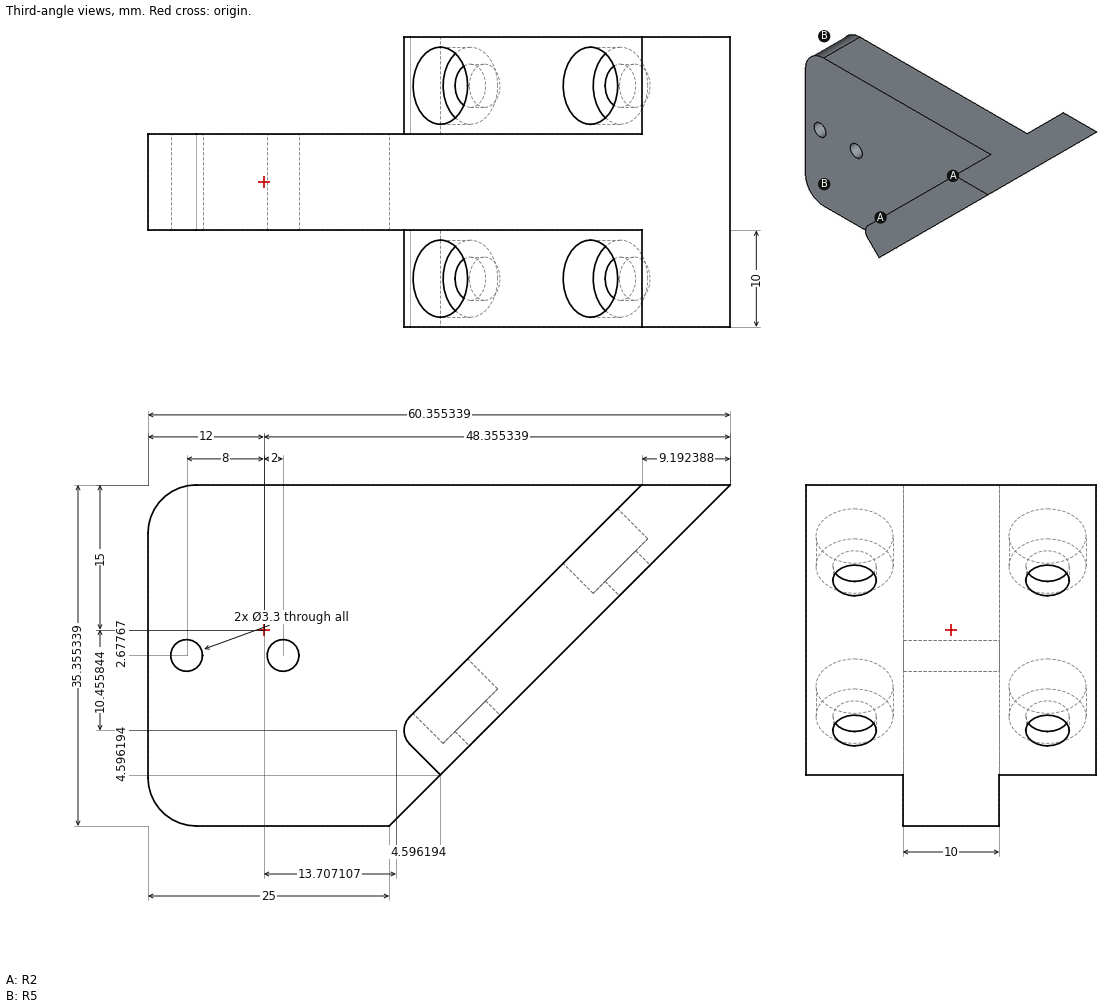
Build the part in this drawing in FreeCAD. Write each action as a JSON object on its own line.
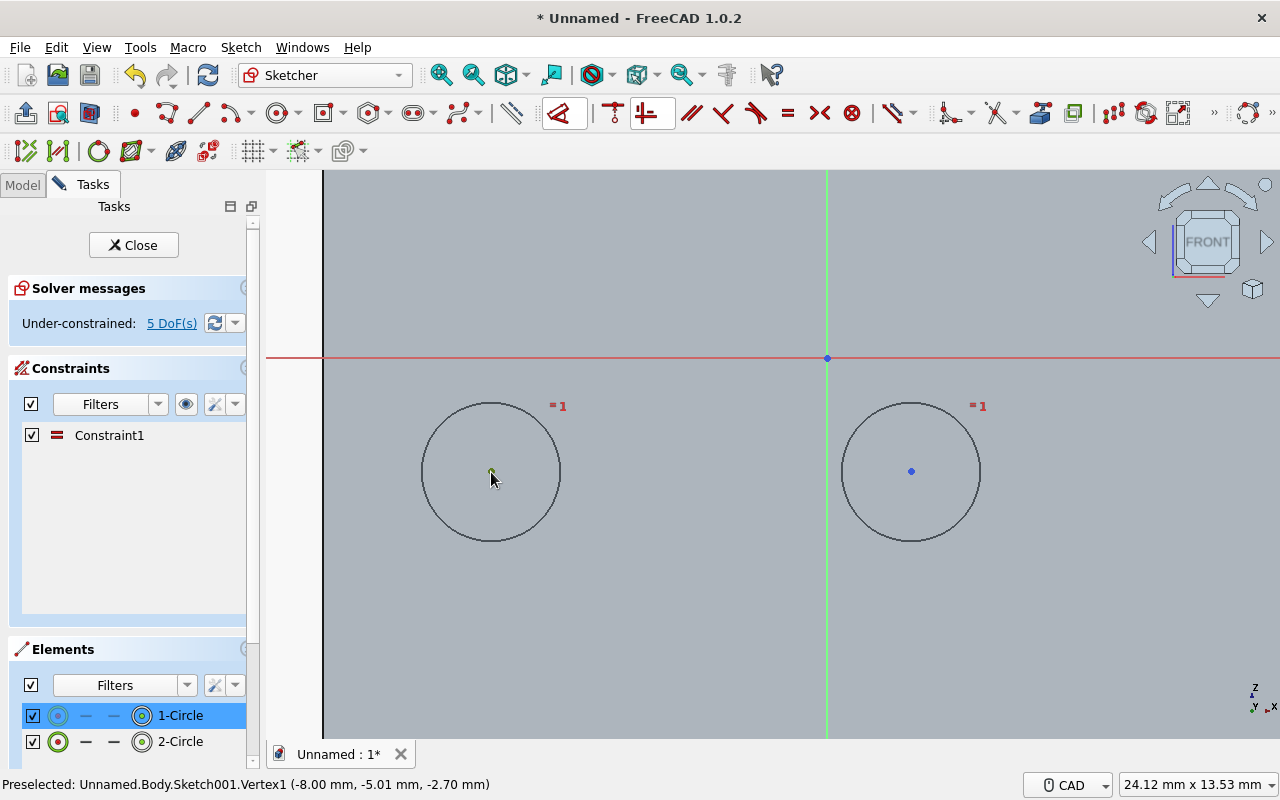
{"action": "left_click", "coordinate": [911, 472]}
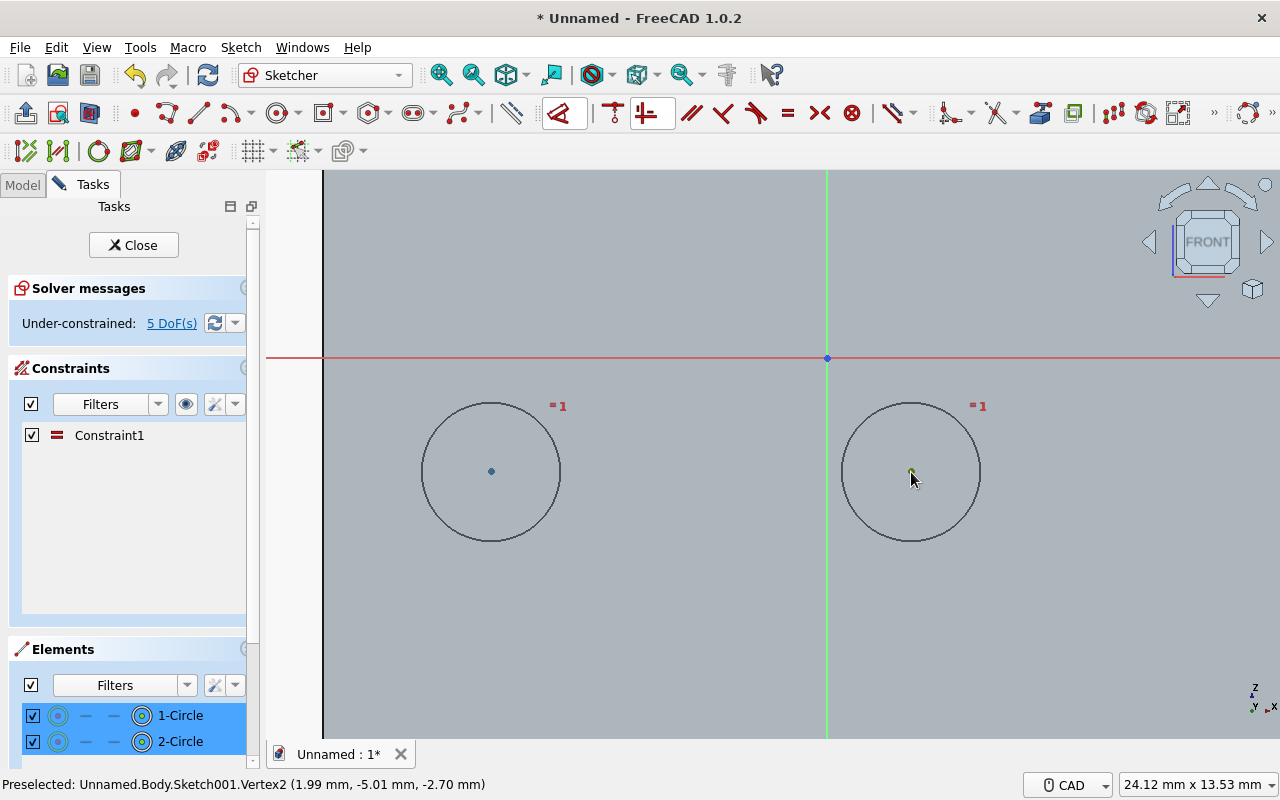
{"action": "left_click", "coordinate": [670, 114]}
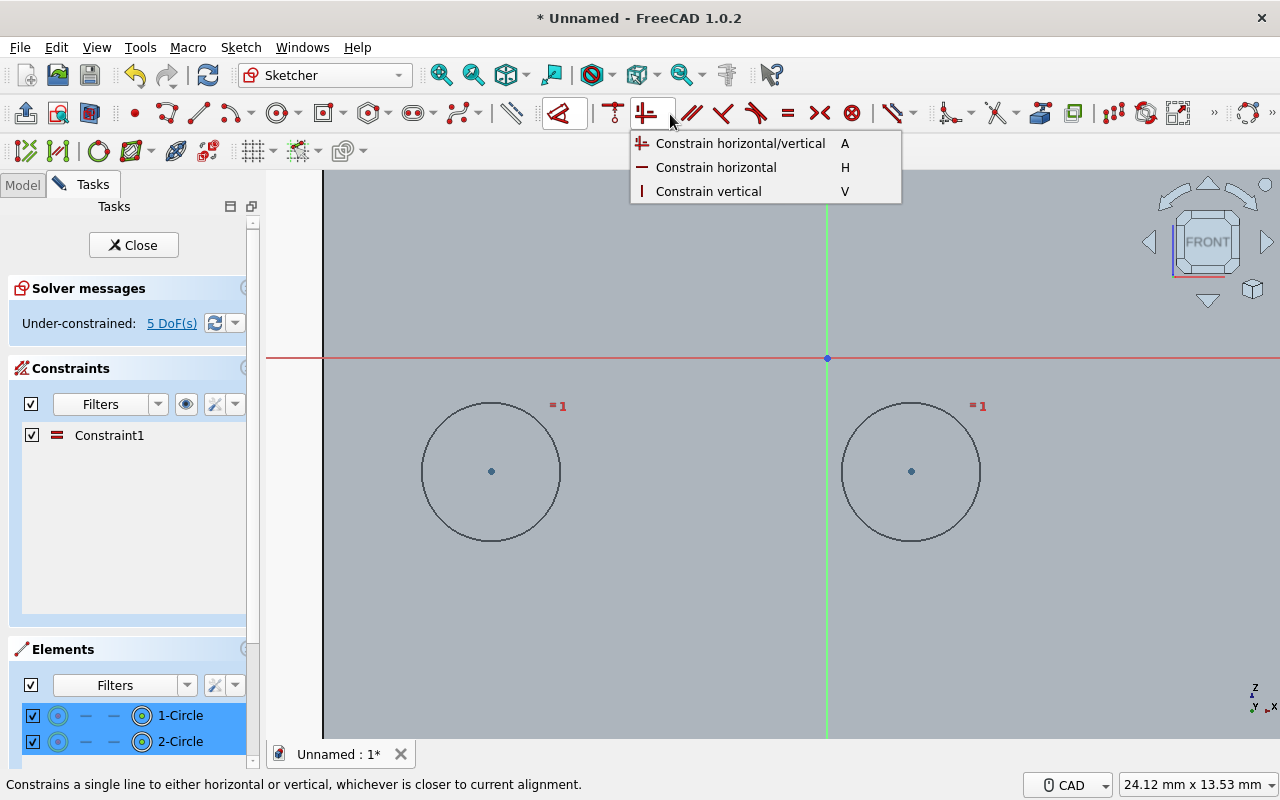
{"action": "left_click", "coordinate": [766, 167]}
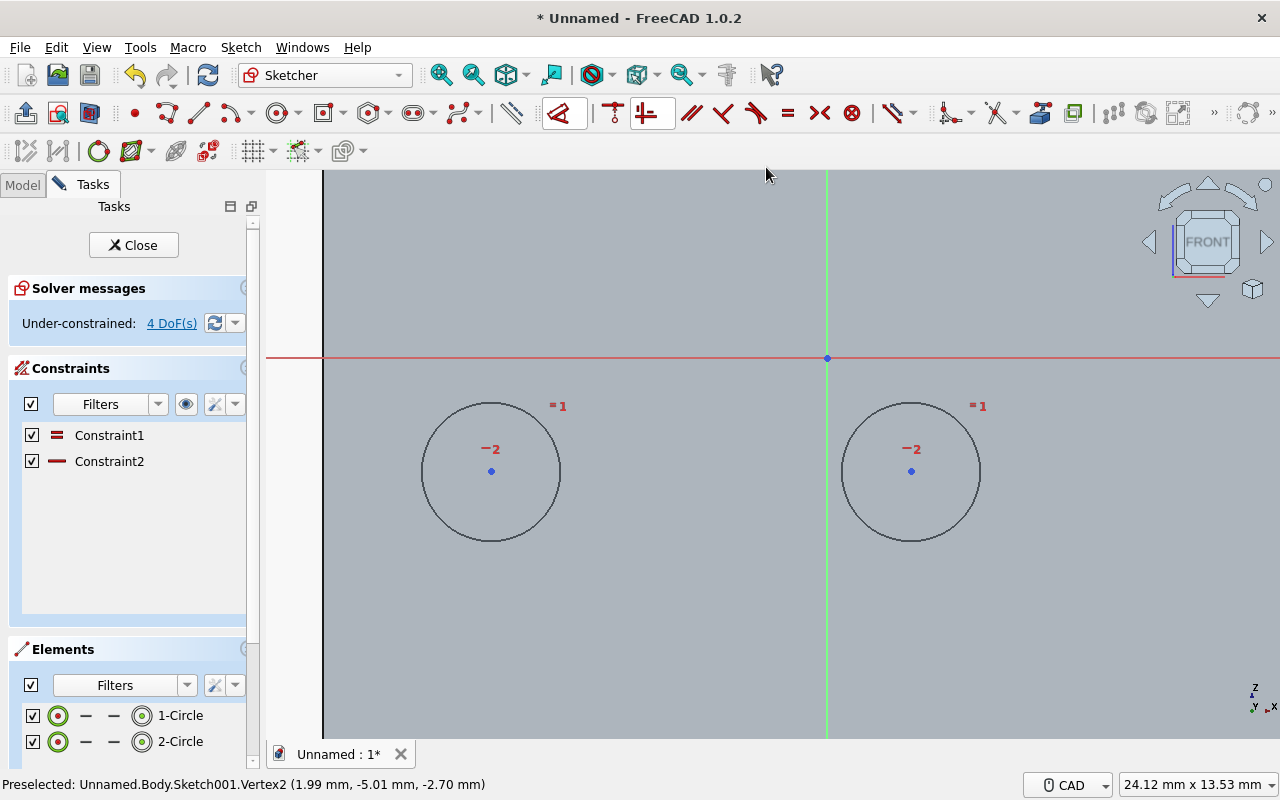
{"action": "left_click", "coordinate": [540, 423]}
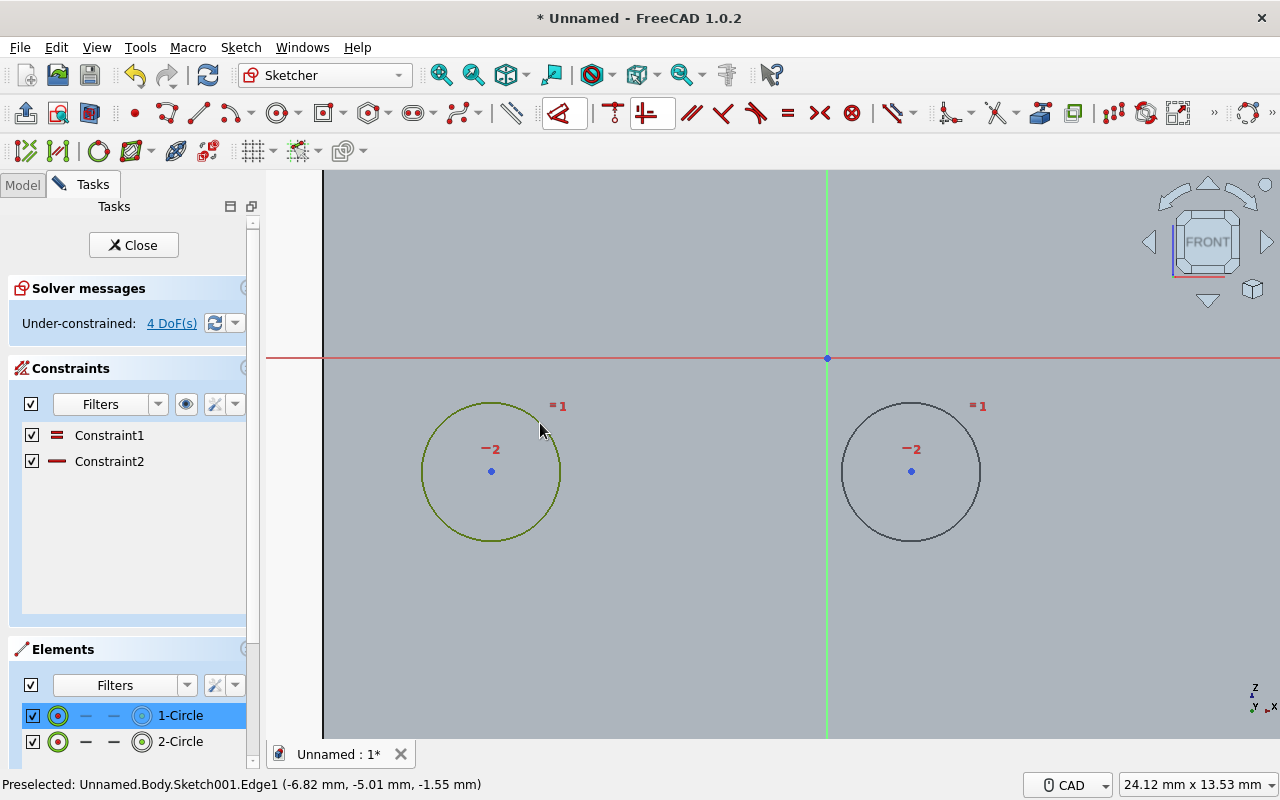
{"action": "left_click", "coordinate": [582, 114]}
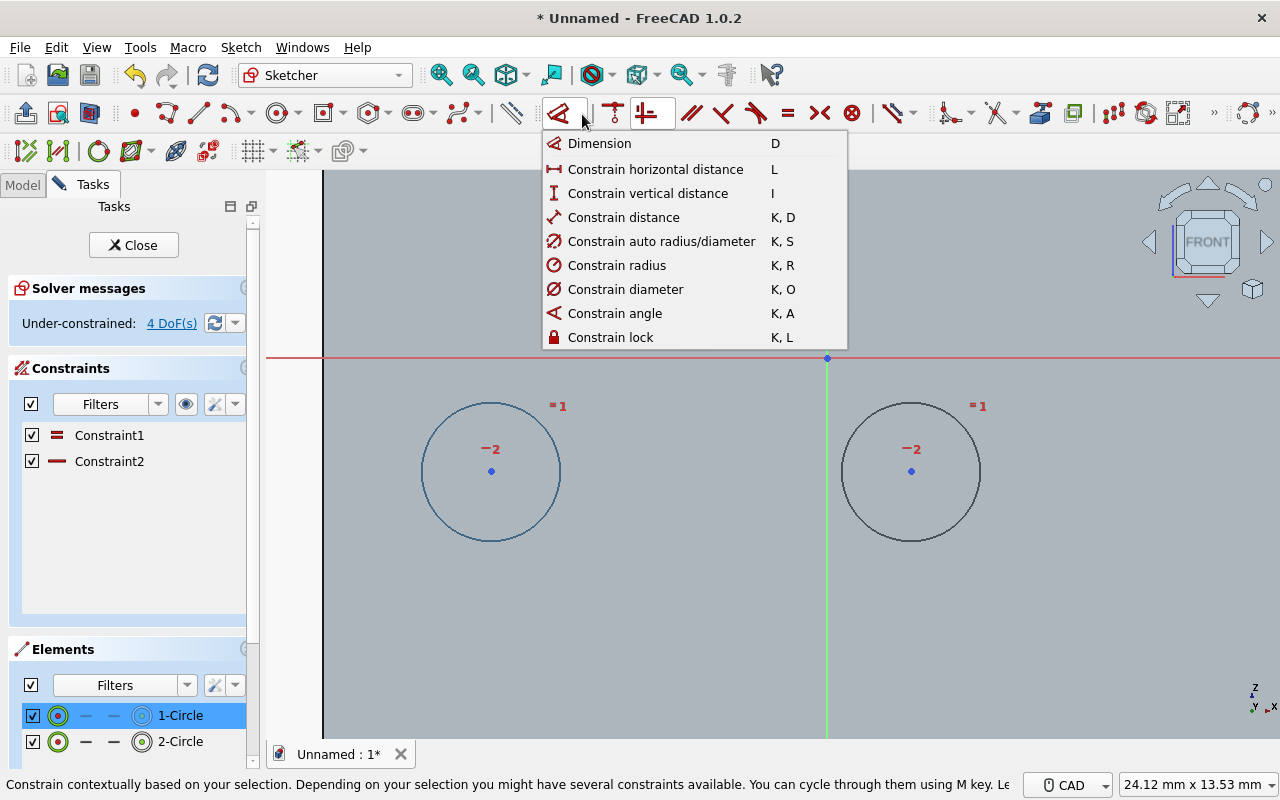
{"action": "left_click", "coordinate": [695, 289]}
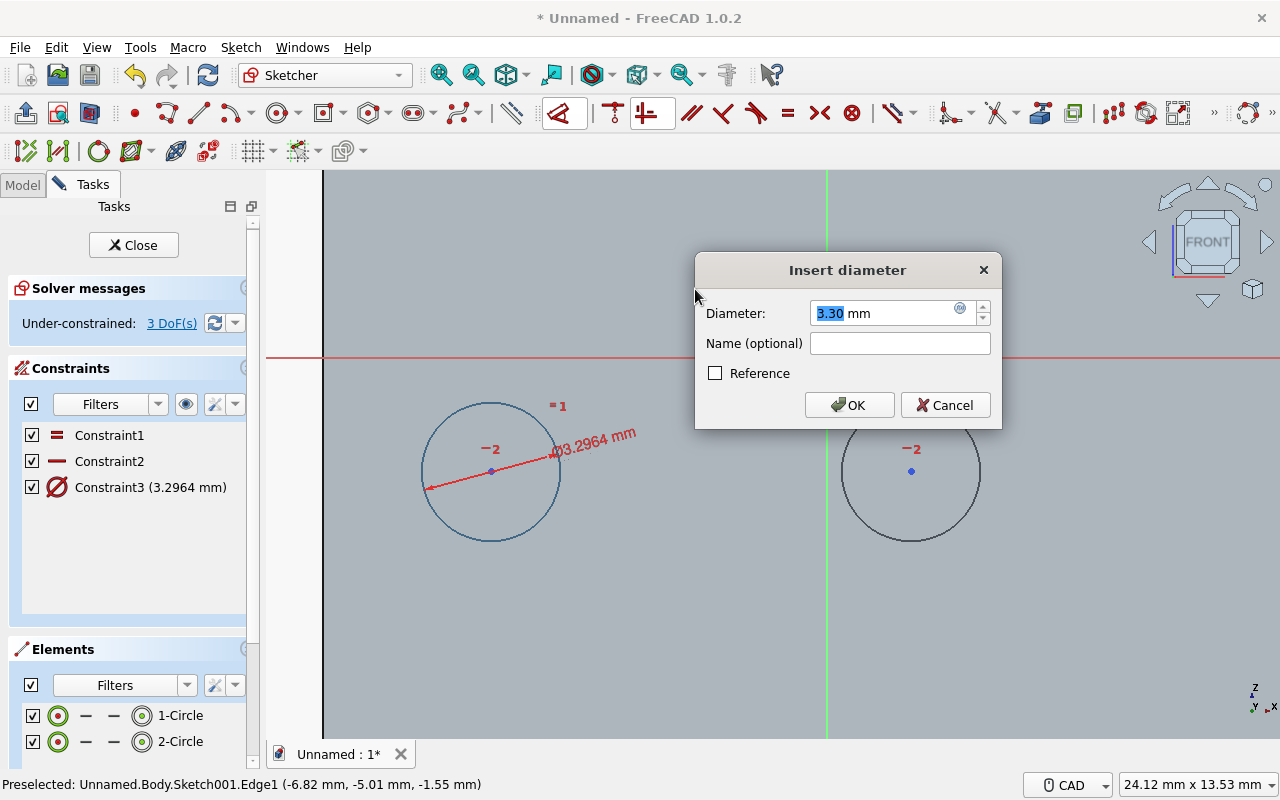
{"action": "type", "text": "3.3"}
{"action": "key", "text": "Return"}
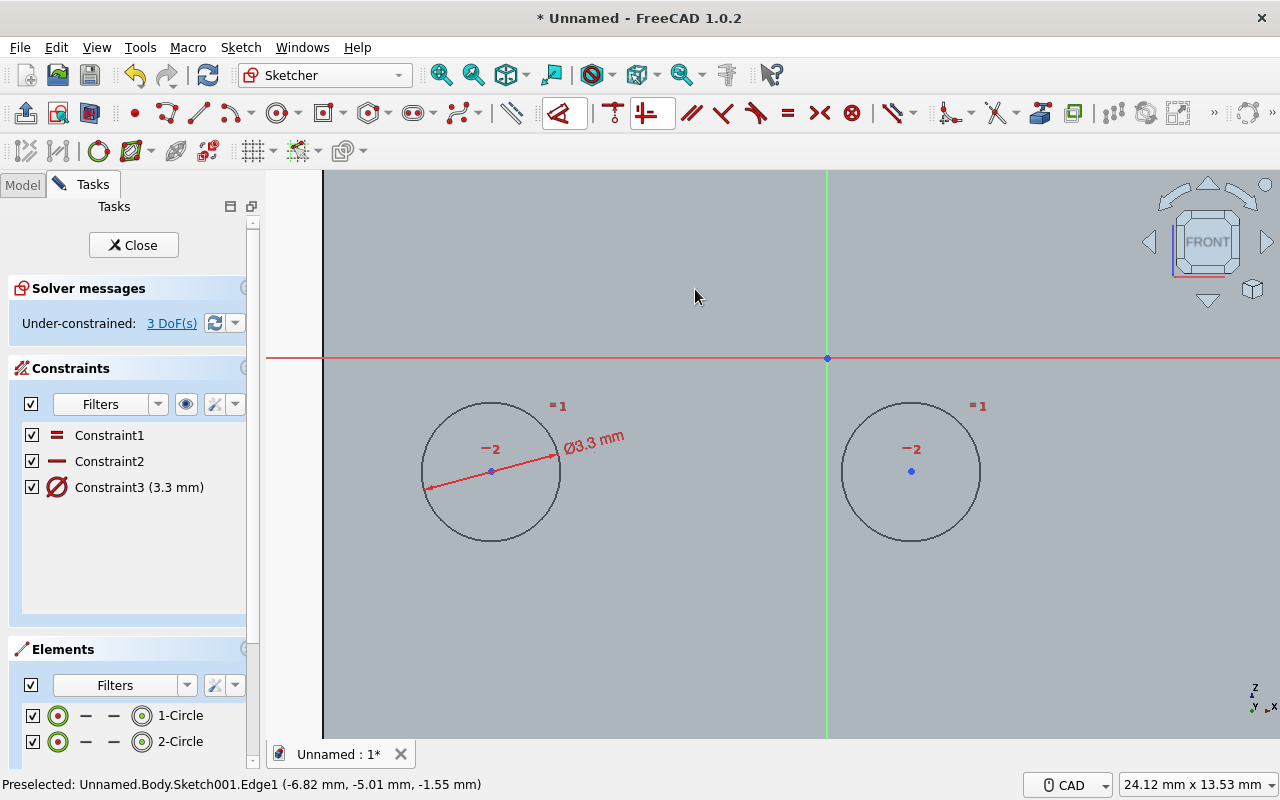
{"action": "left_click", "coordinate": [491, 472]}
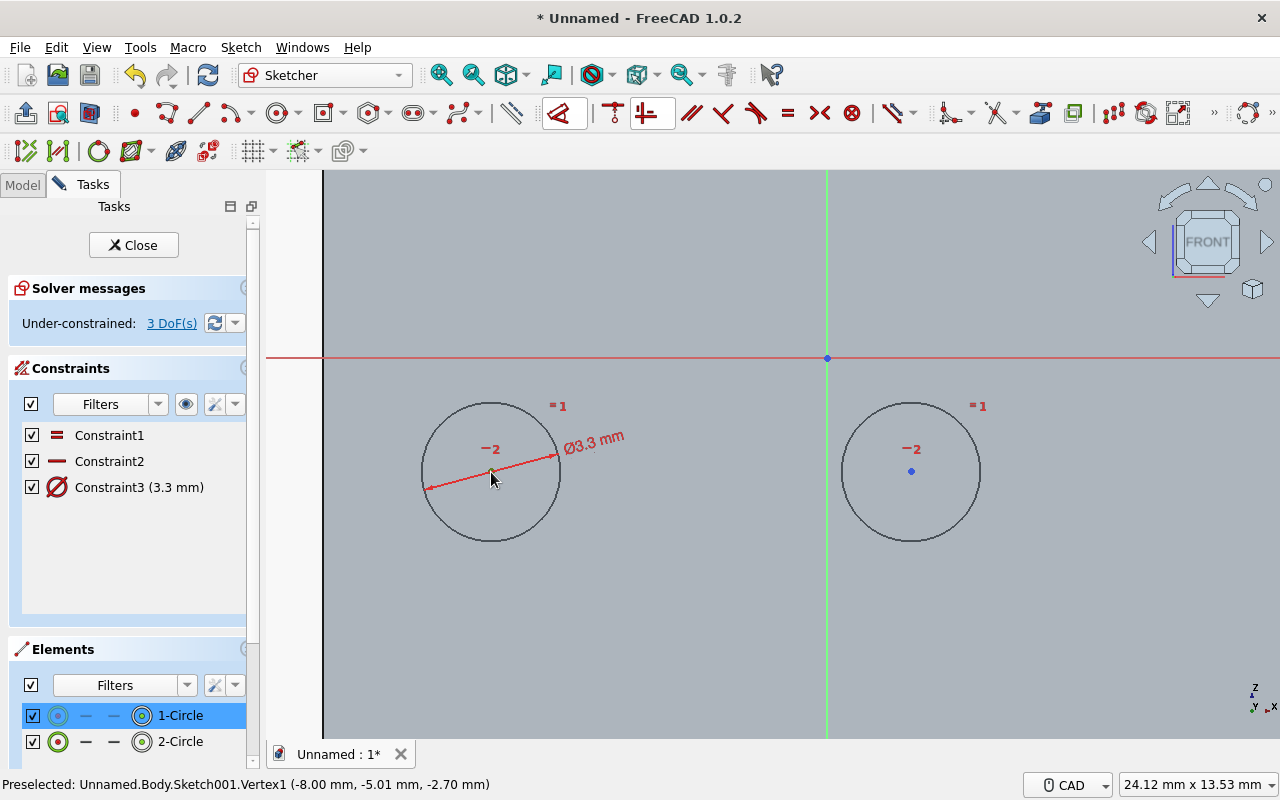
{"action": "left_click", "coordinate": [582, 114]}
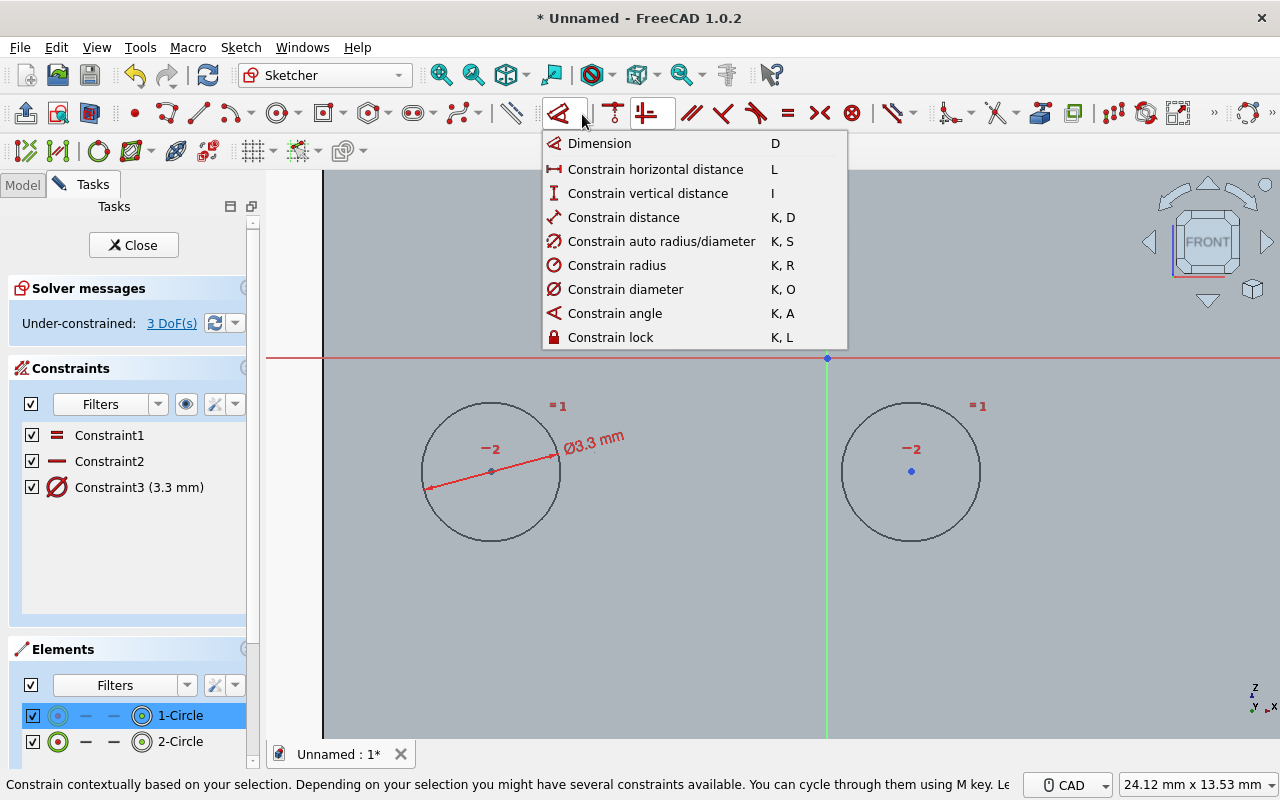
{"action": "left_click", "coordinate": [695, 169]}